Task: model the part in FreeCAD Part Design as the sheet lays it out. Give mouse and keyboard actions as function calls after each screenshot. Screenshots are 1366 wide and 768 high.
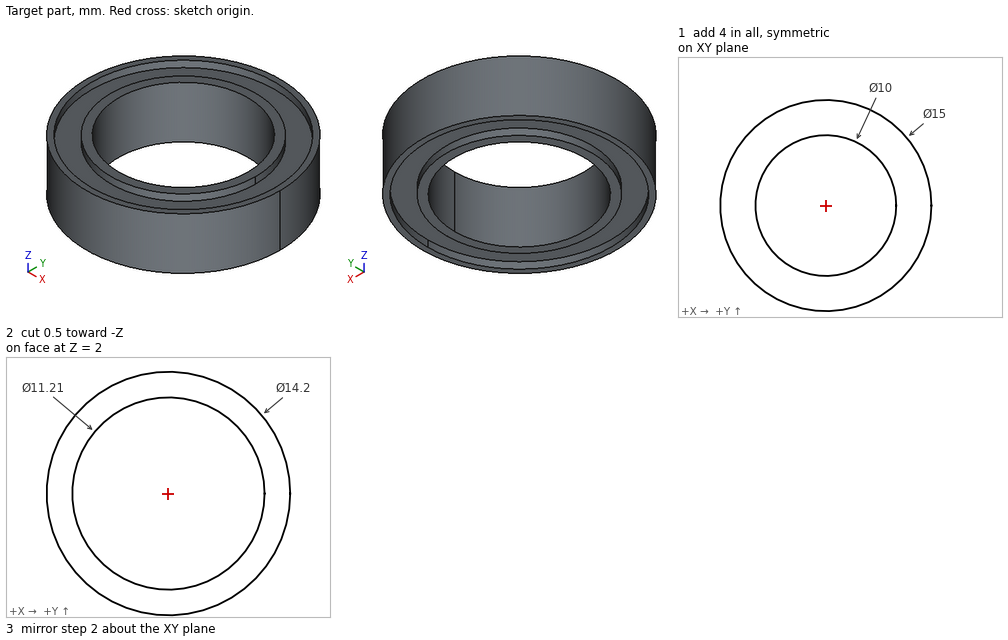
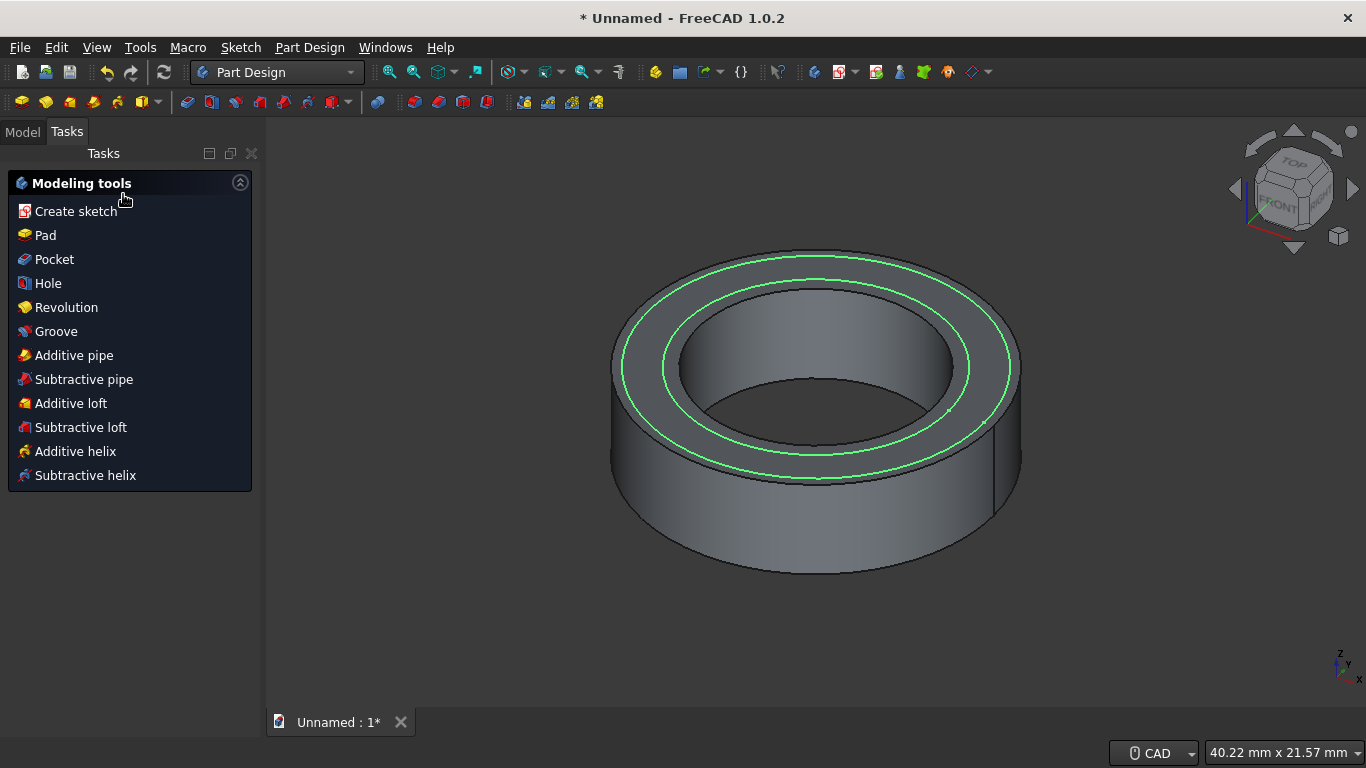
click(188, 102)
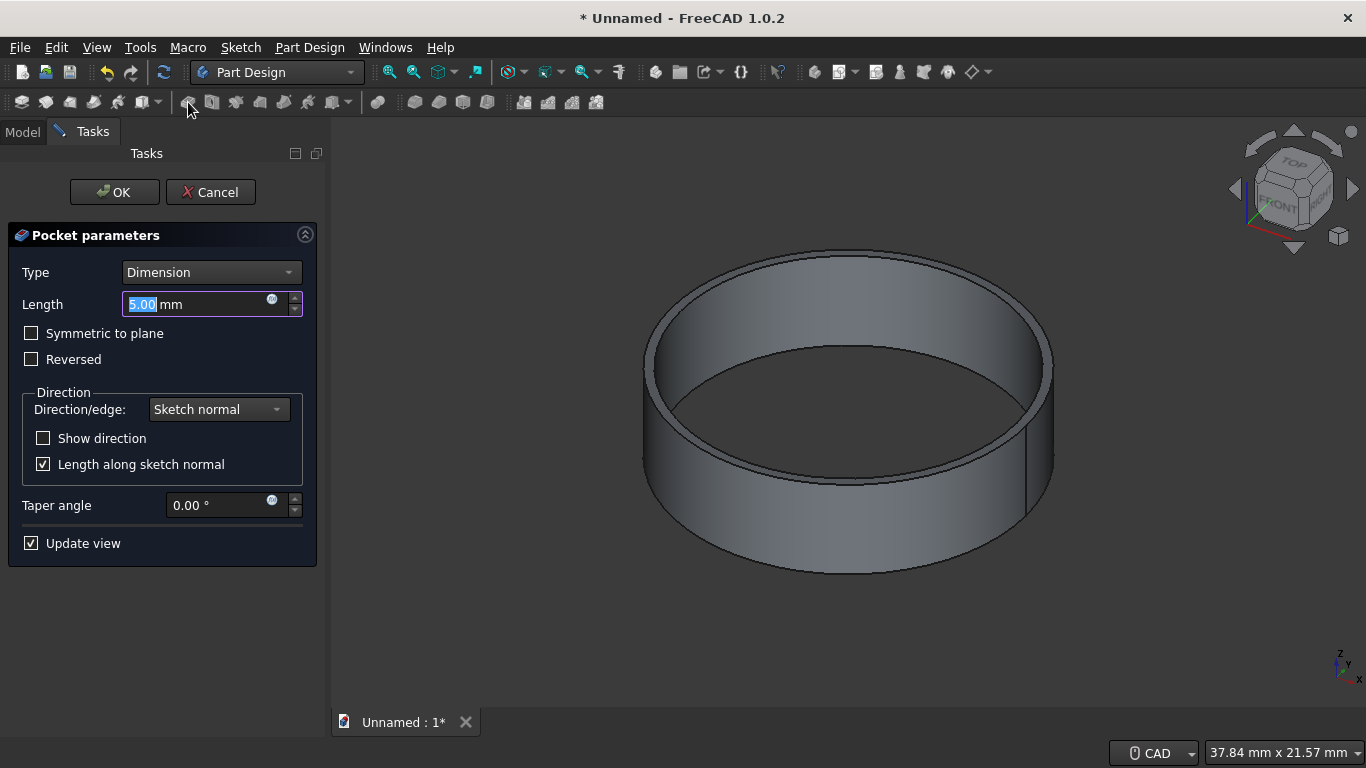
text(0.5)
key(Tab)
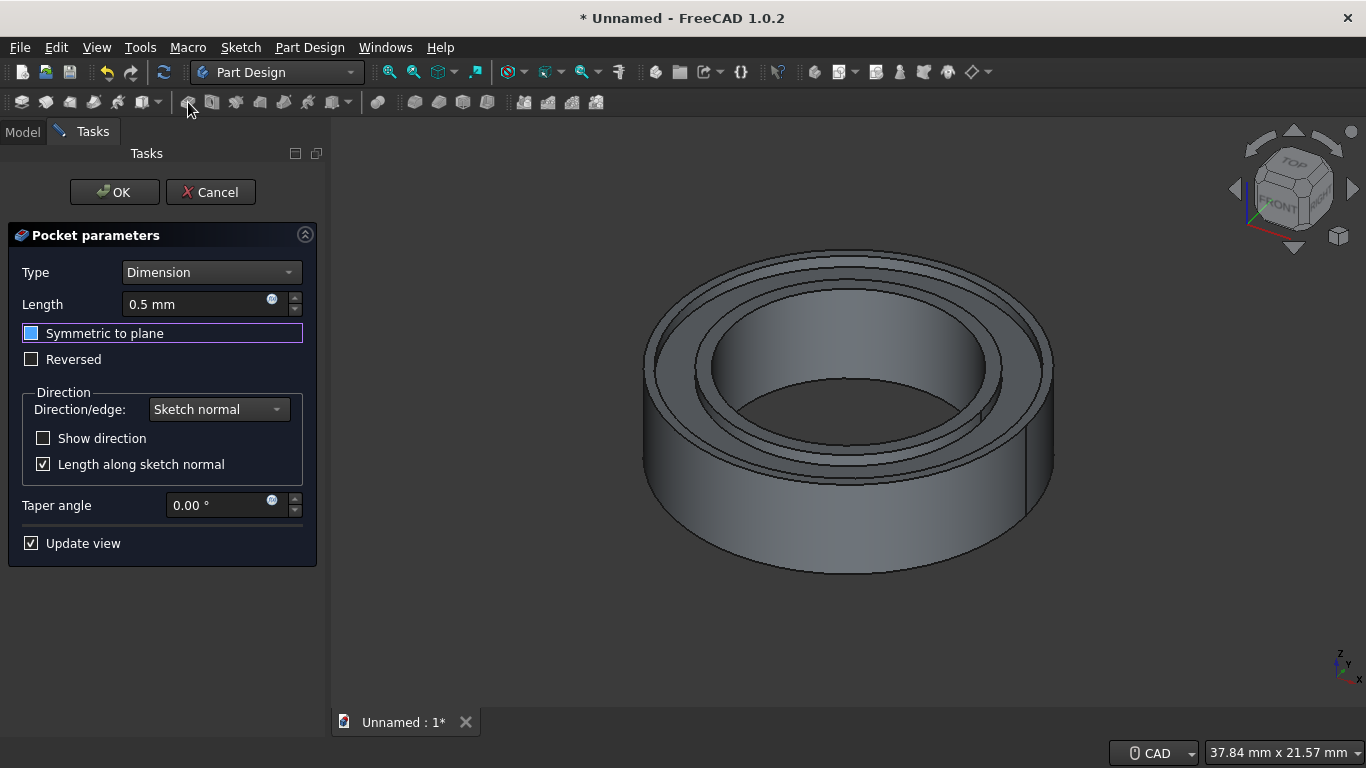
click(115, 192)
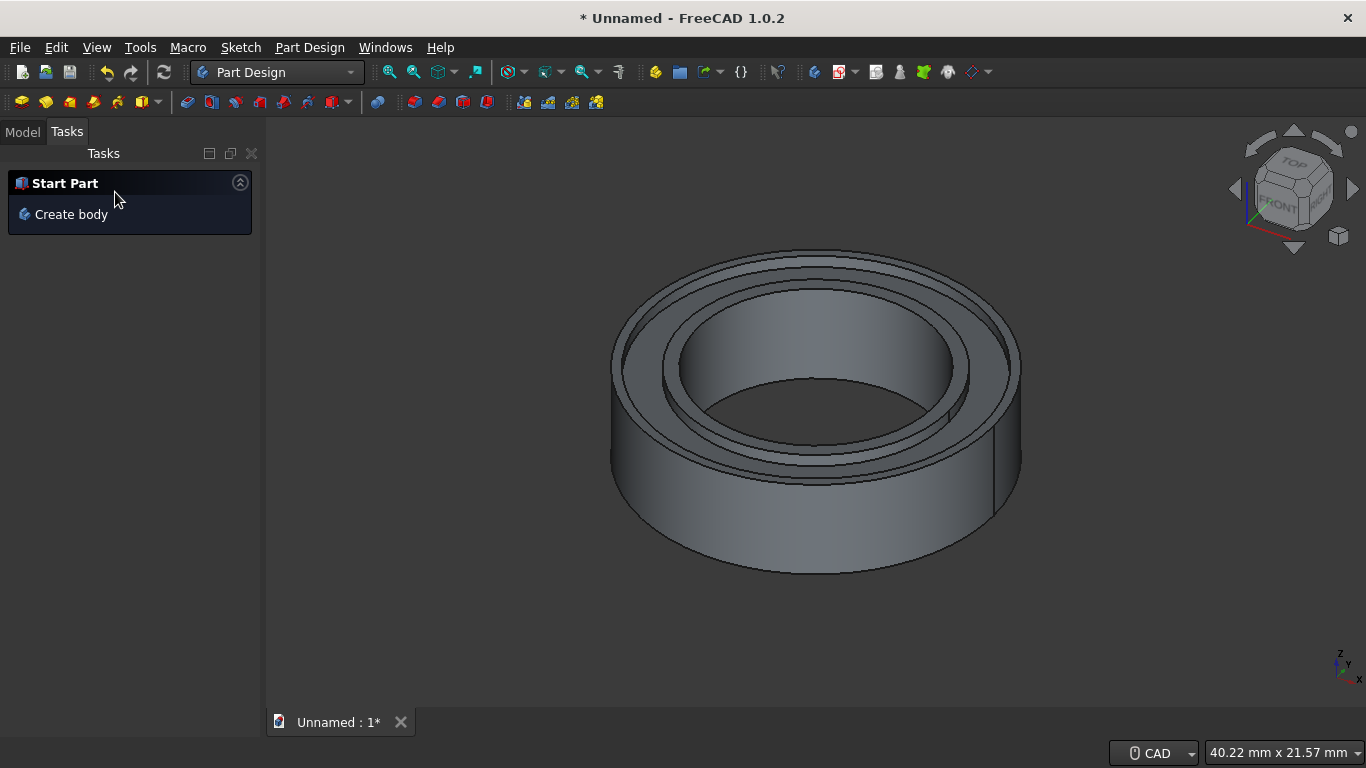
click(23, 131)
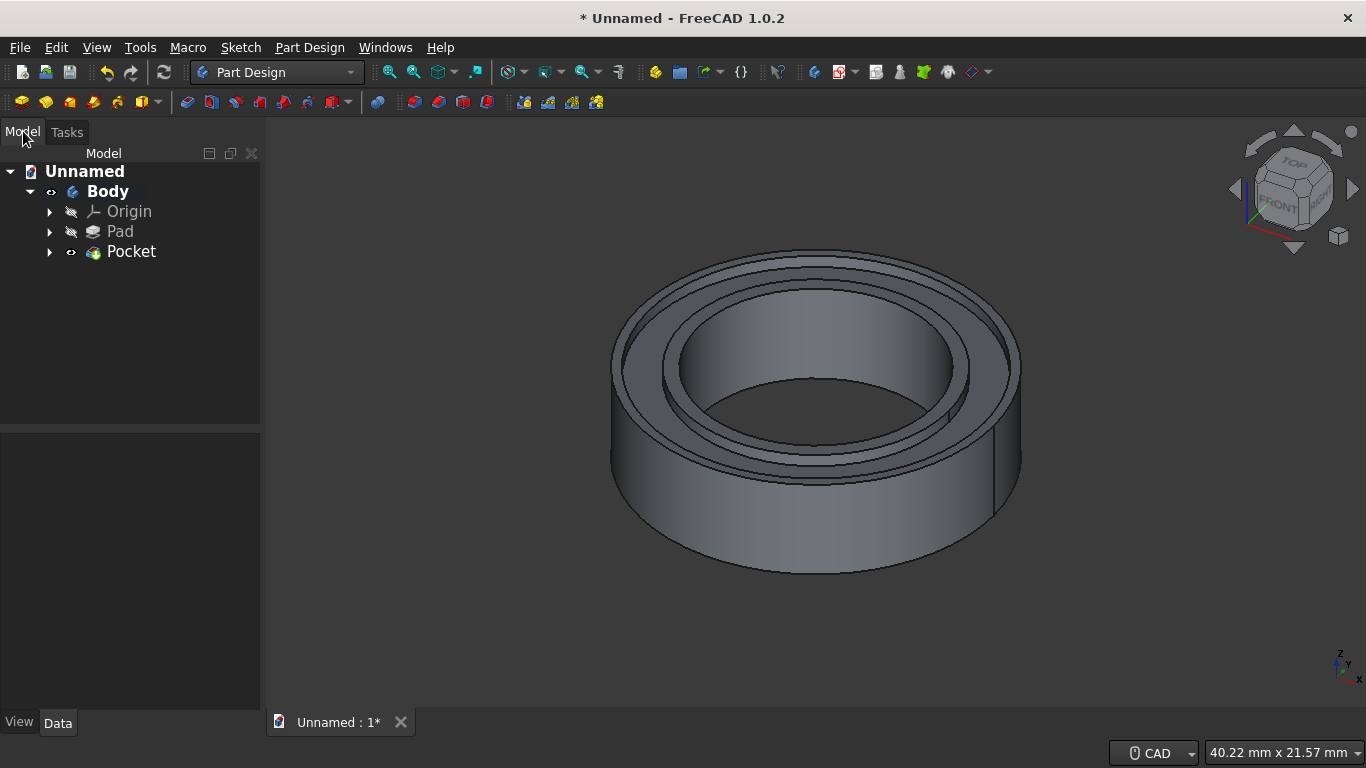
click(116, 252)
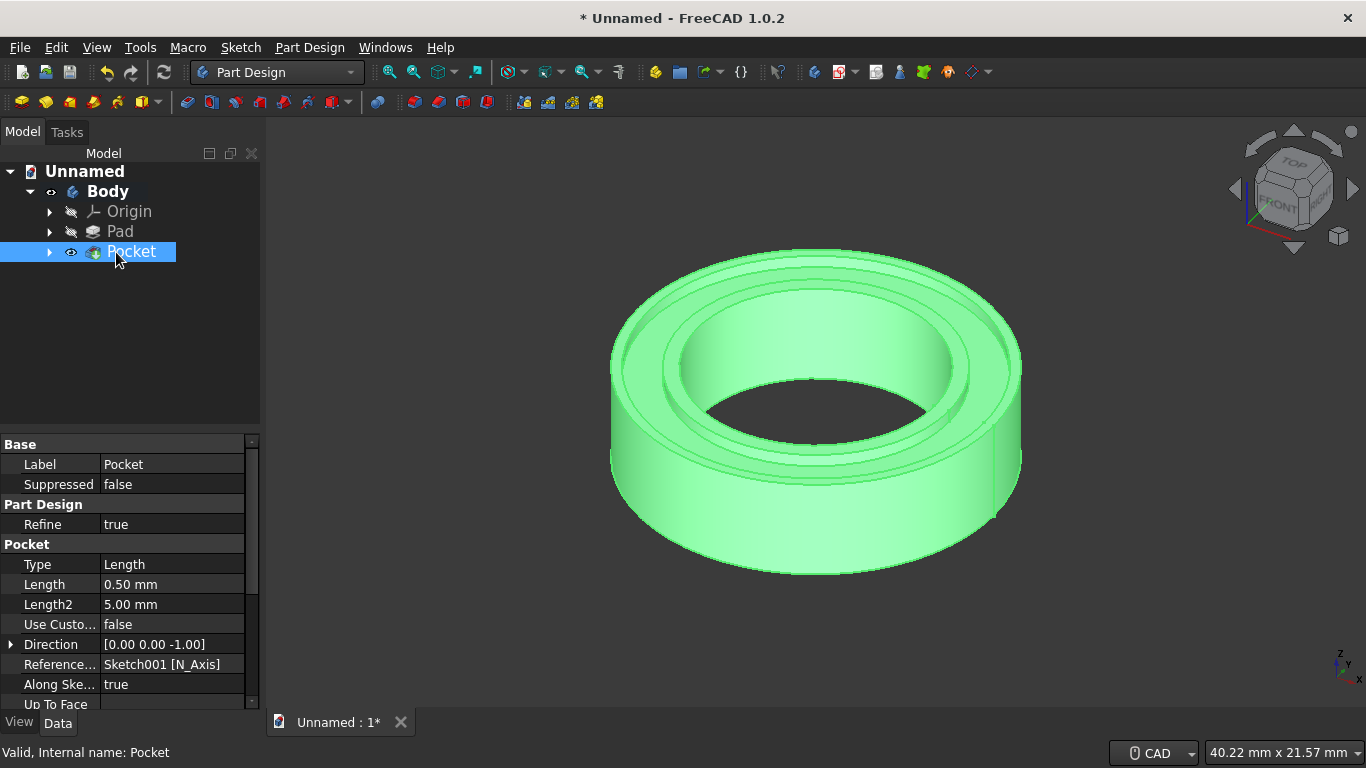
click(524, 102)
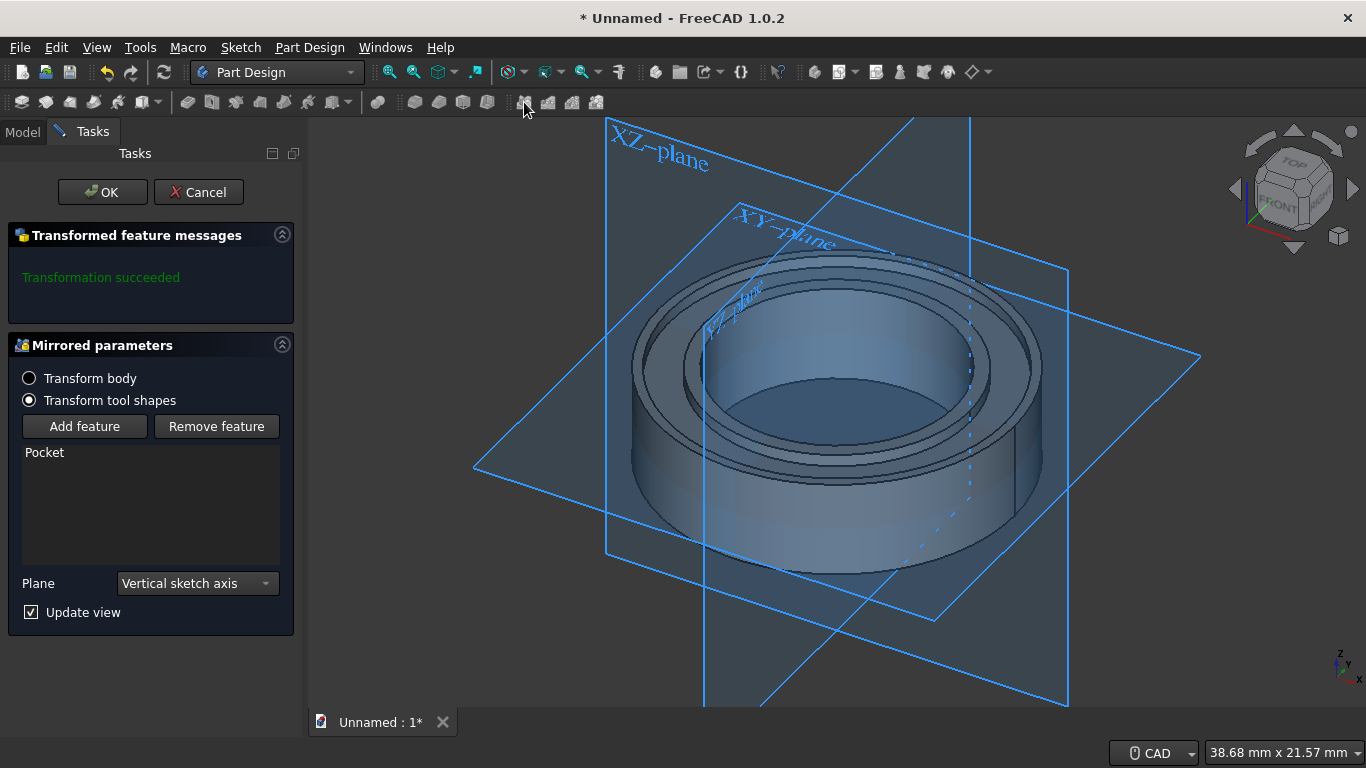
click(198, 584)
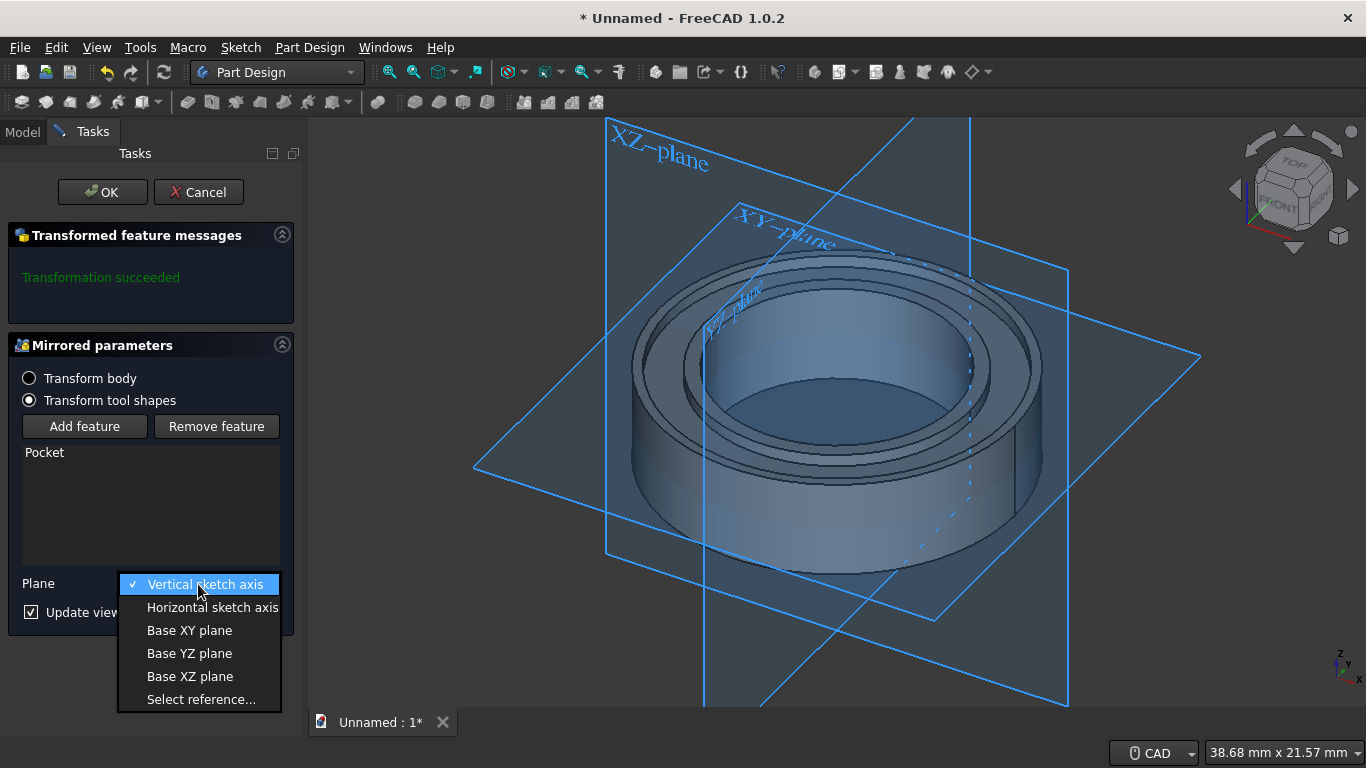
click(198, 630)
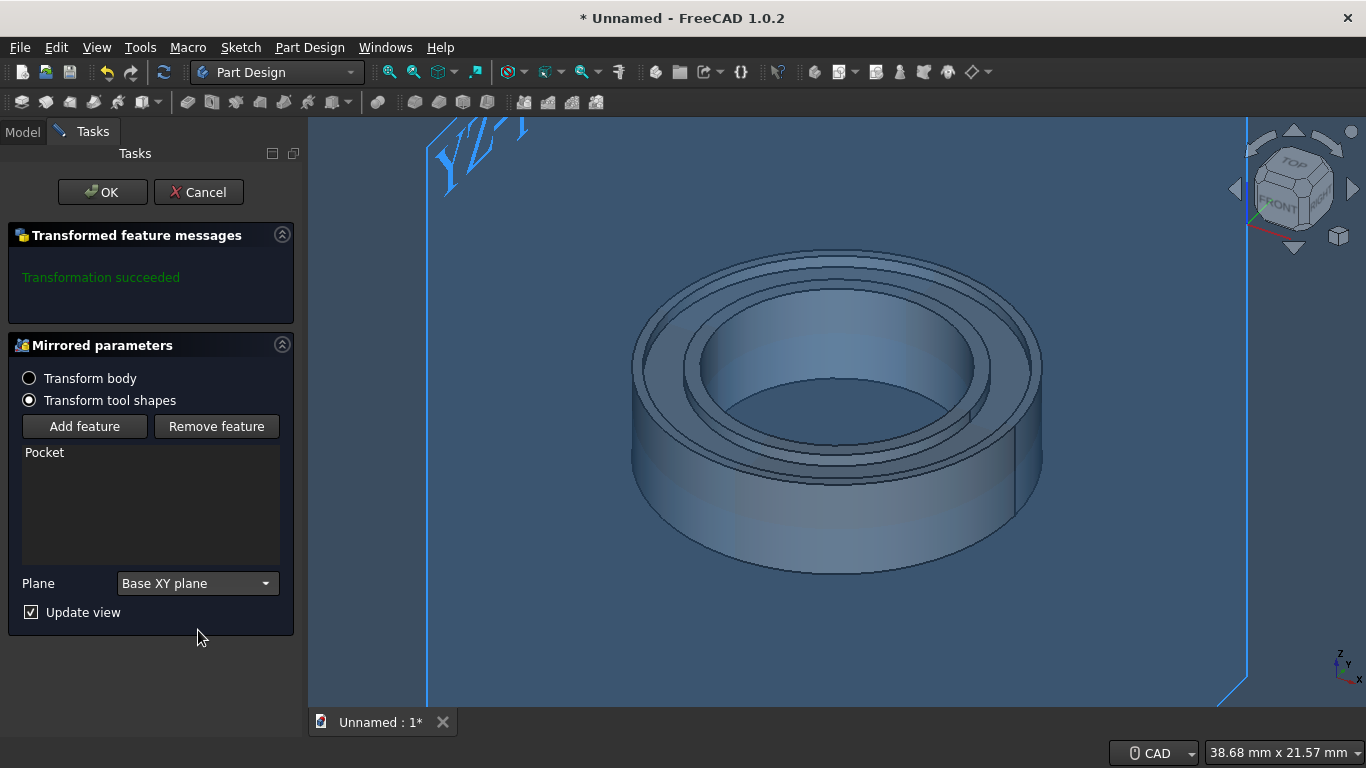
click(103, 192)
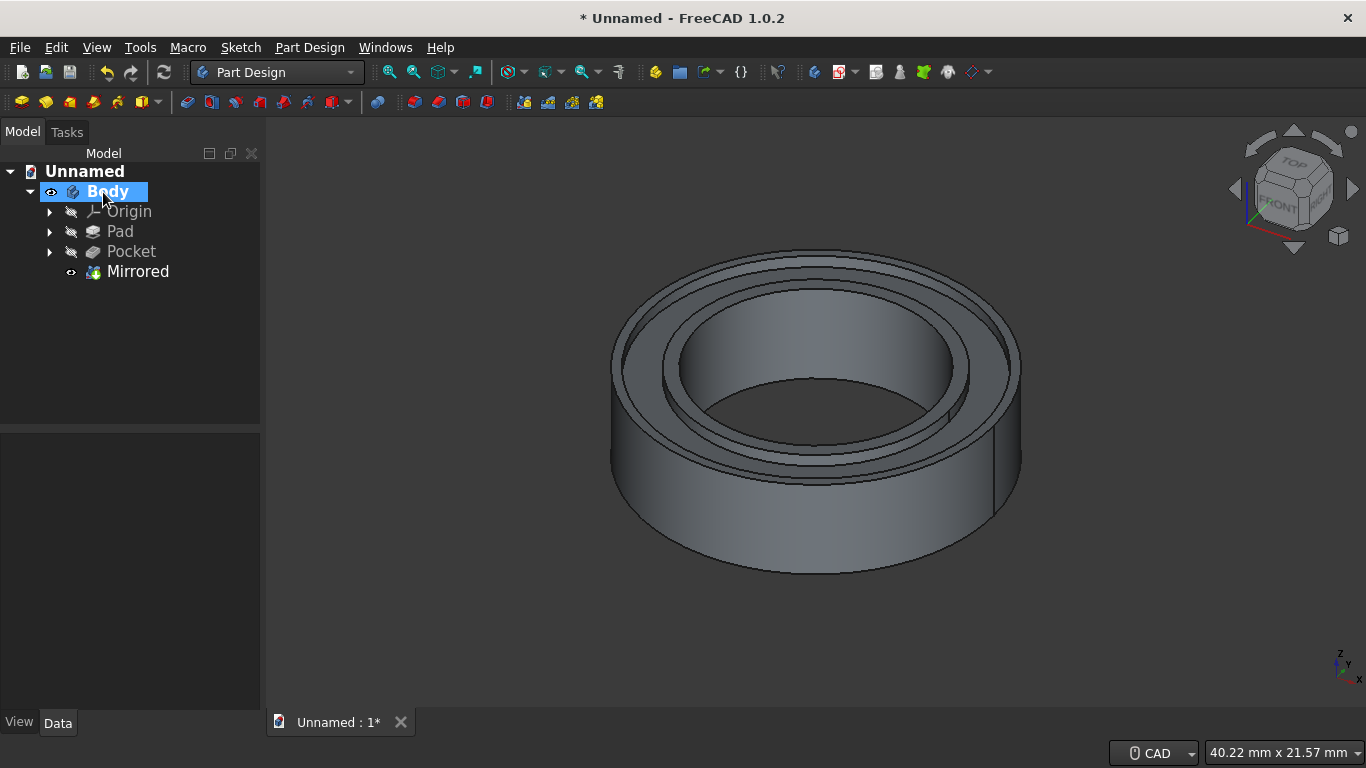
key(0)